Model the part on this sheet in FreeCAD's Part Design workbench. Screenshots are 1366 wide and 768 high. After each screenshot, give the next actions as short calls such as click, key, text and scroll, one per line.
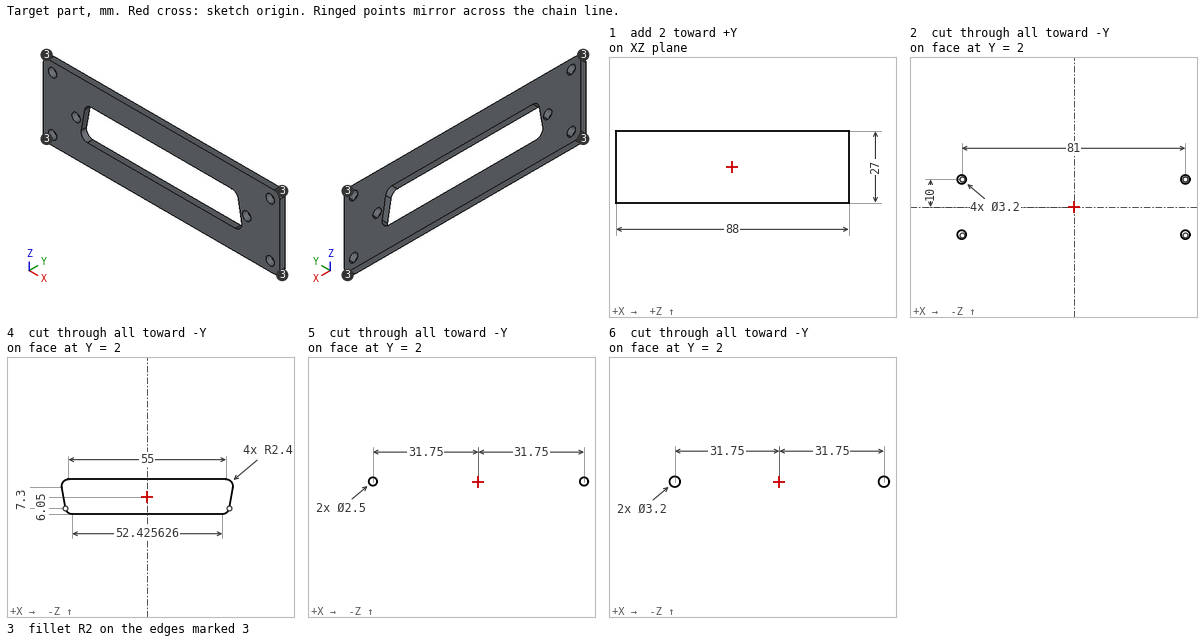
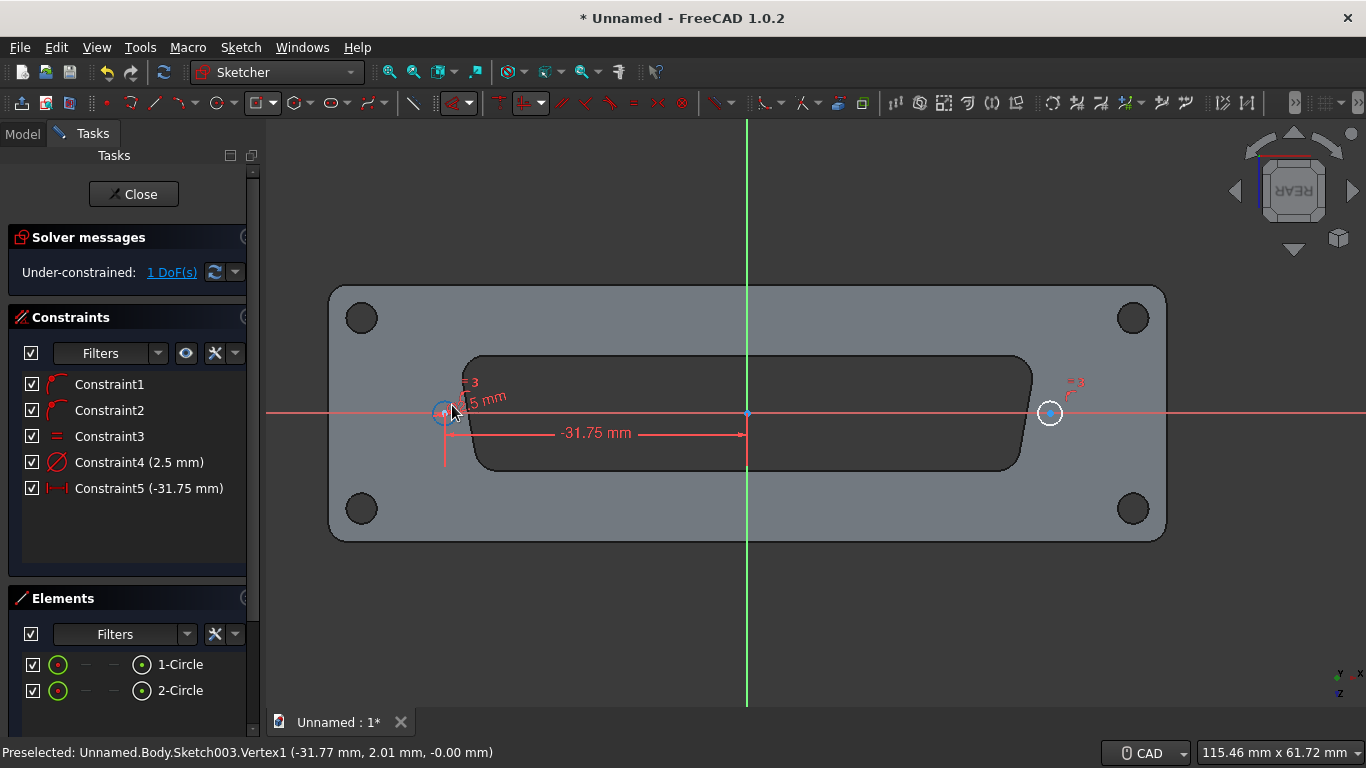
click(1050, 413)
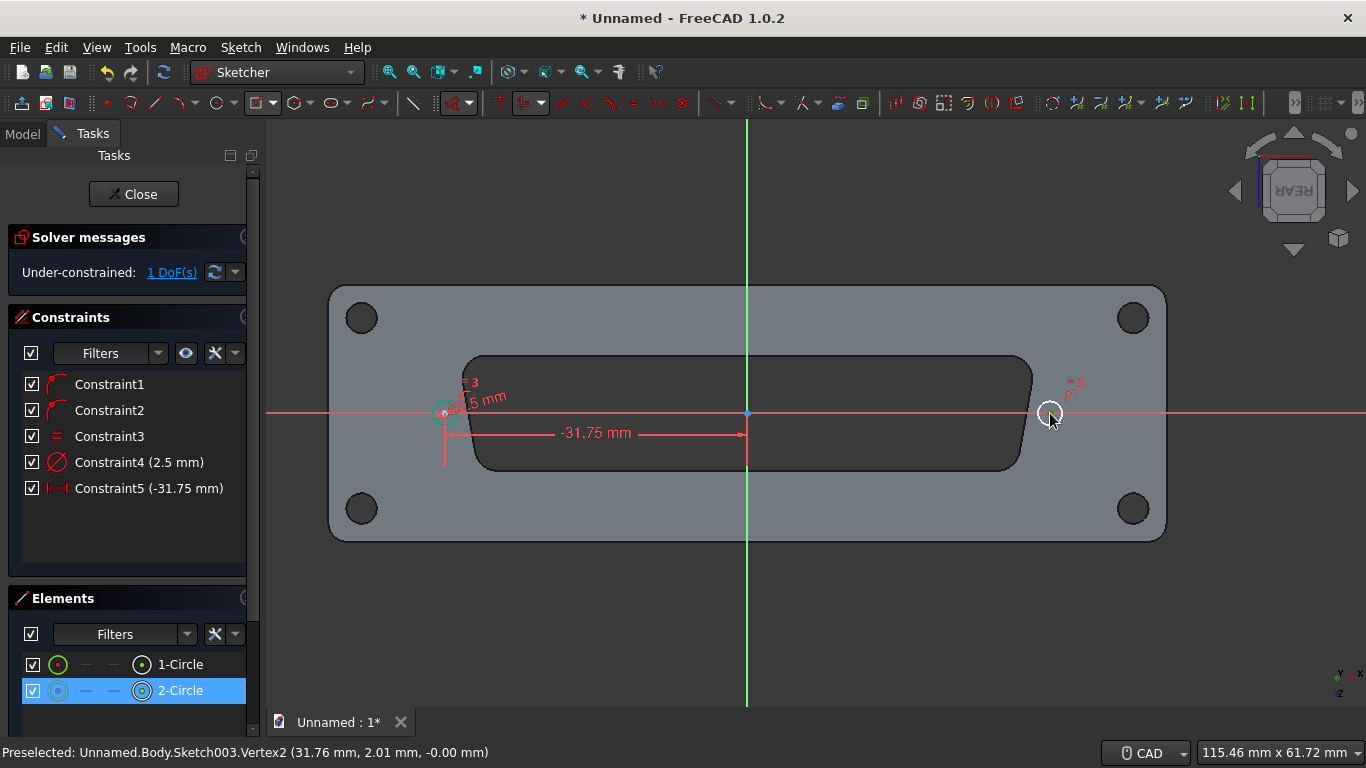
click(472, 104)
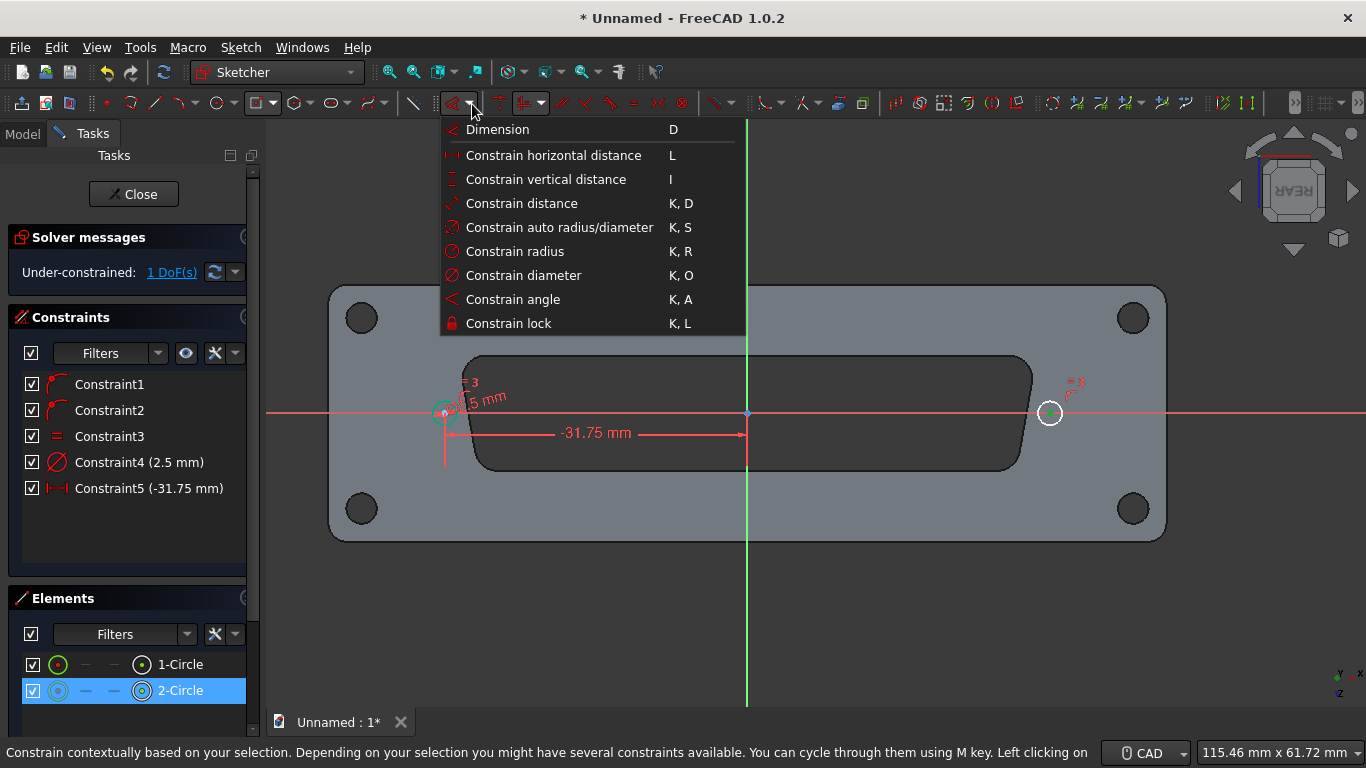
click(593, 155)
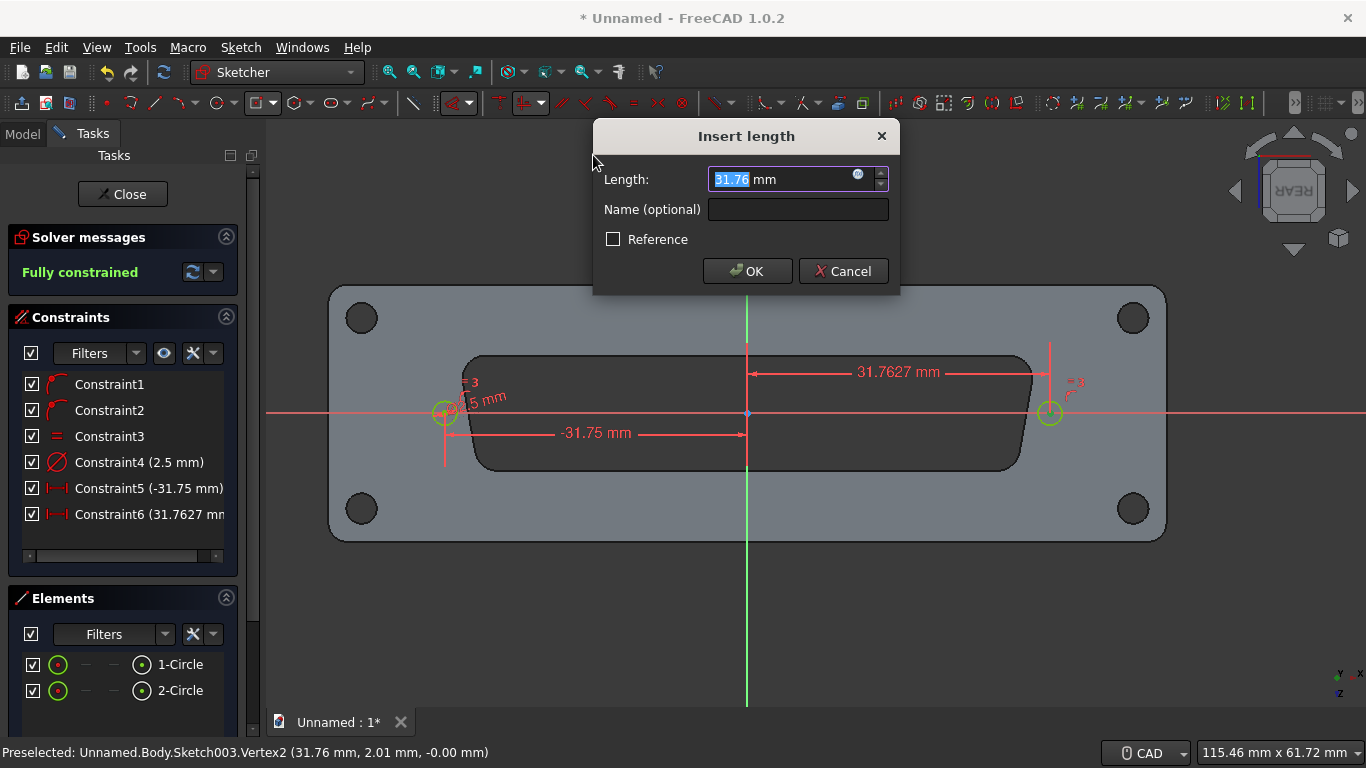
text(31.75)
key(Return)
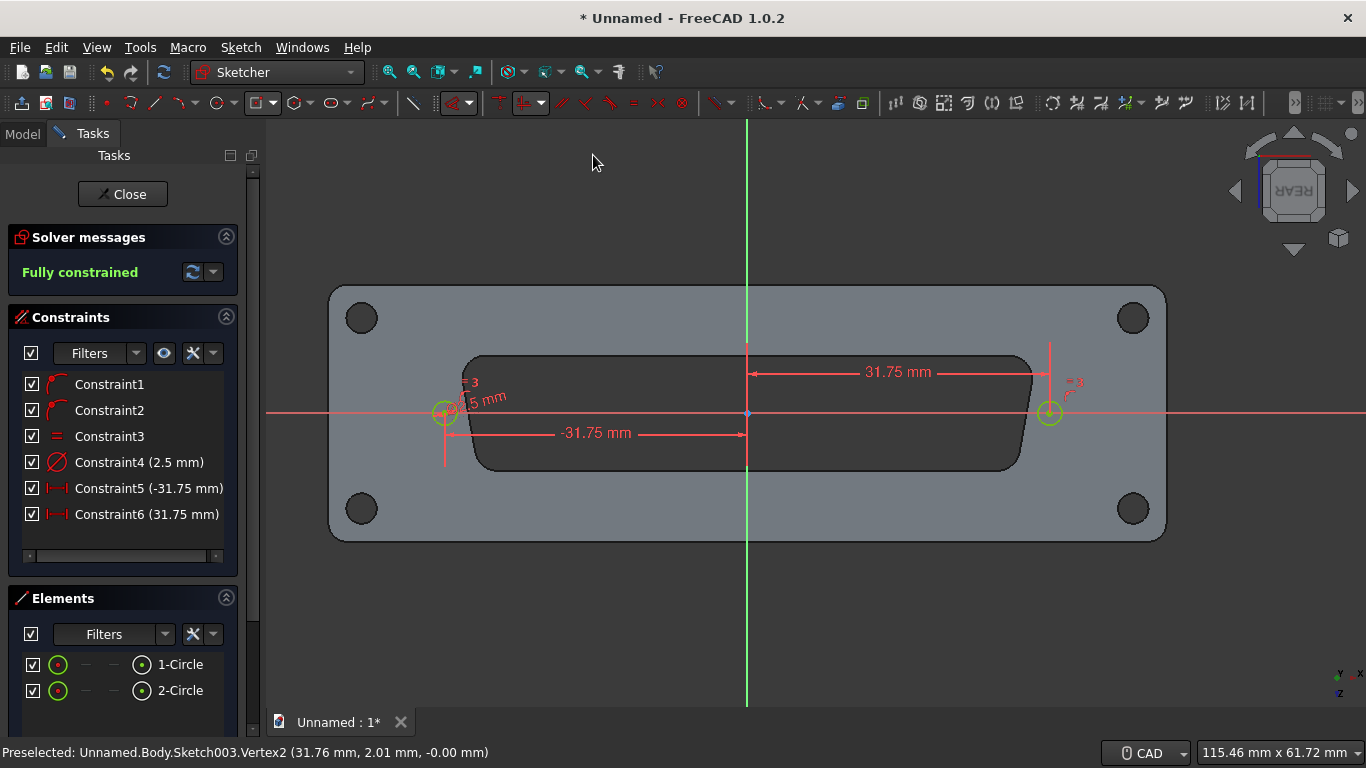
click(123, 194)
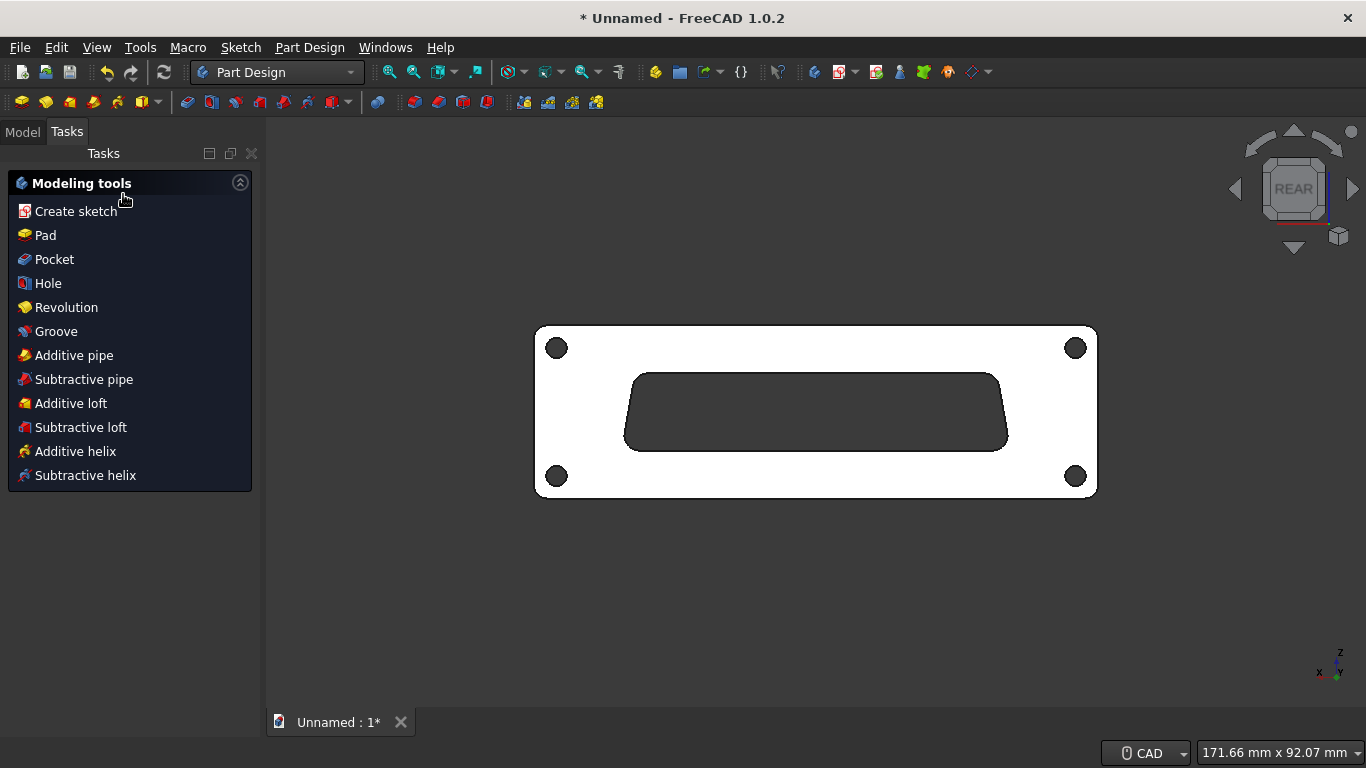
click(188, 102)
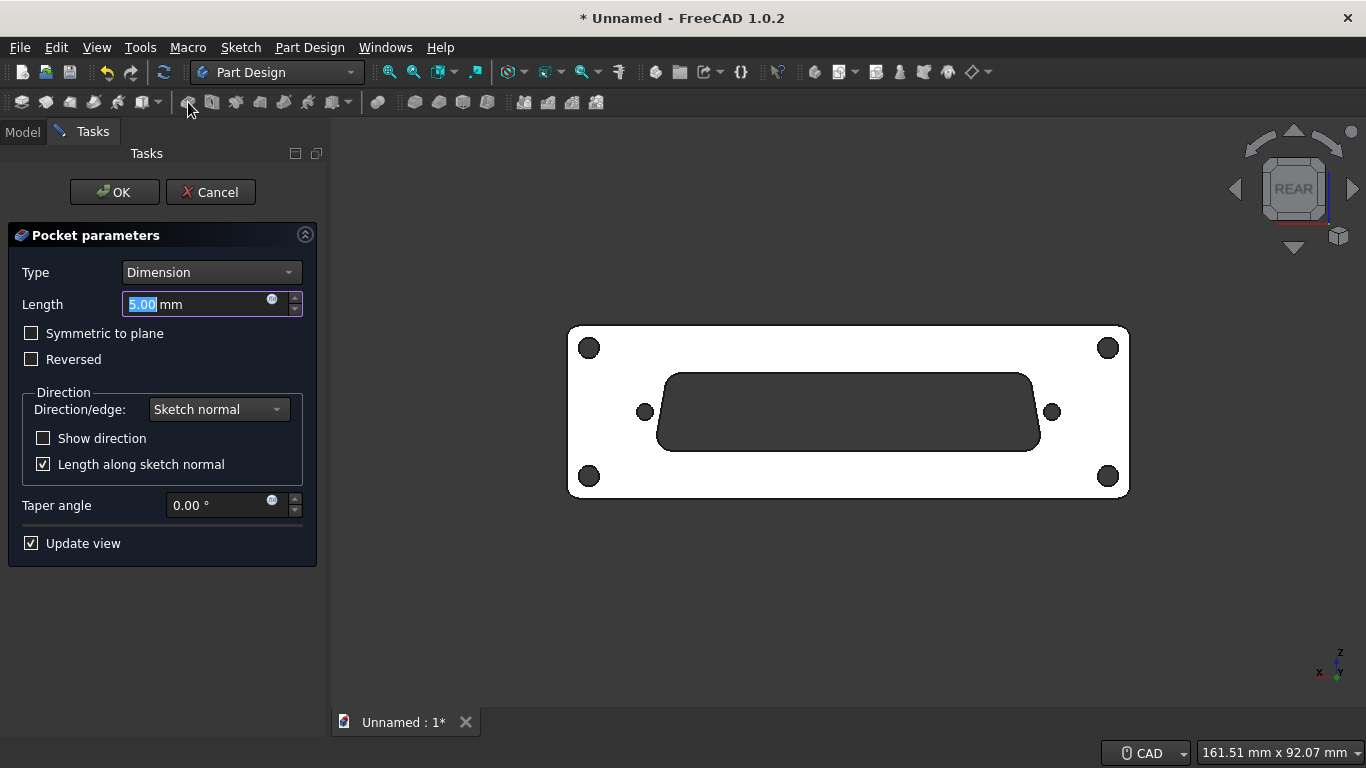
click(212, 272)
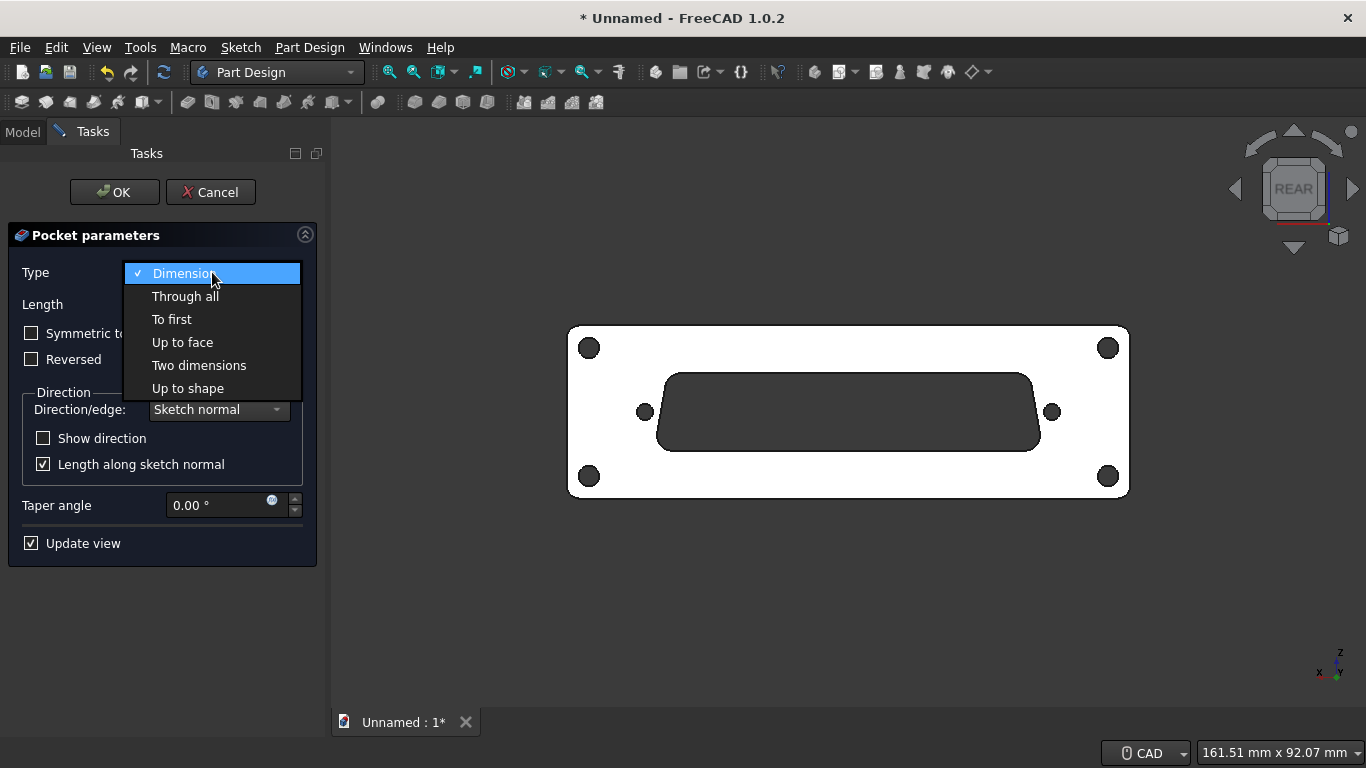
click(212, 296)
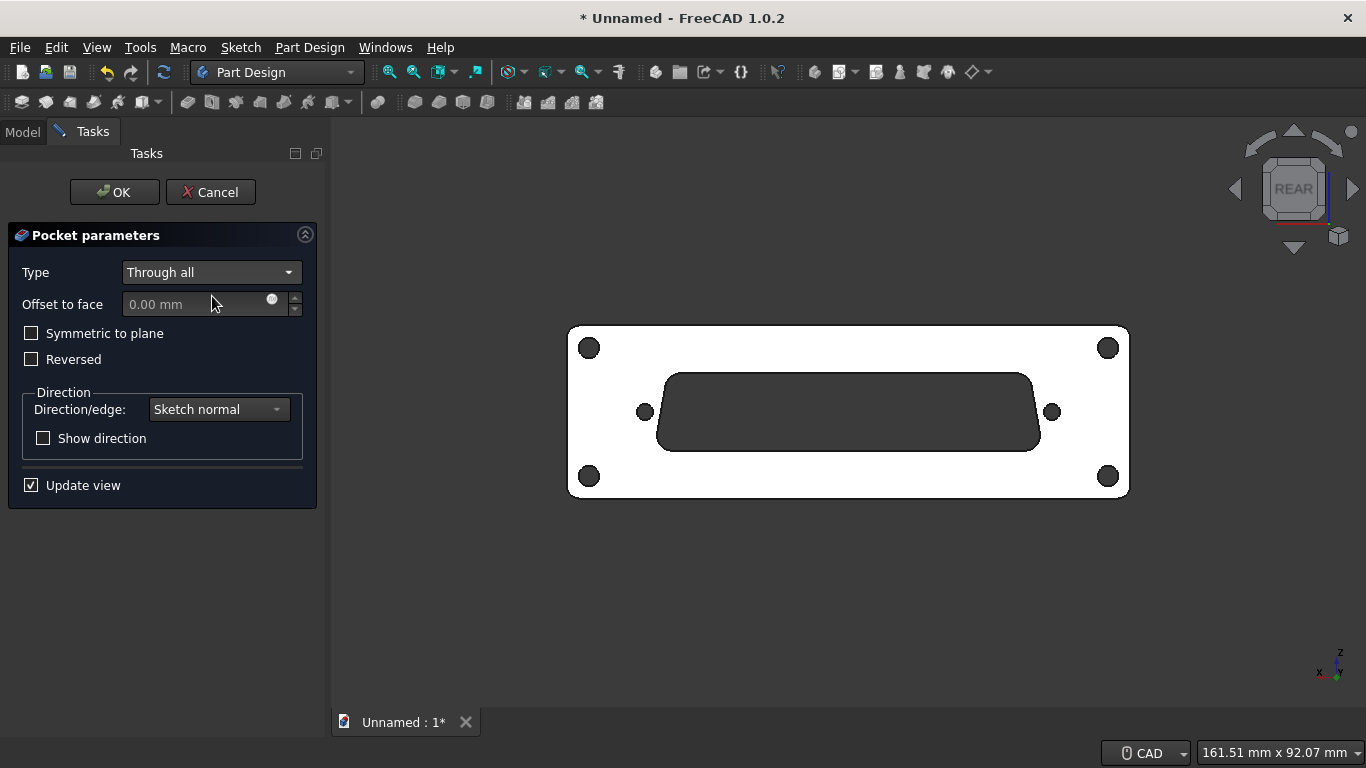
click(115, 192)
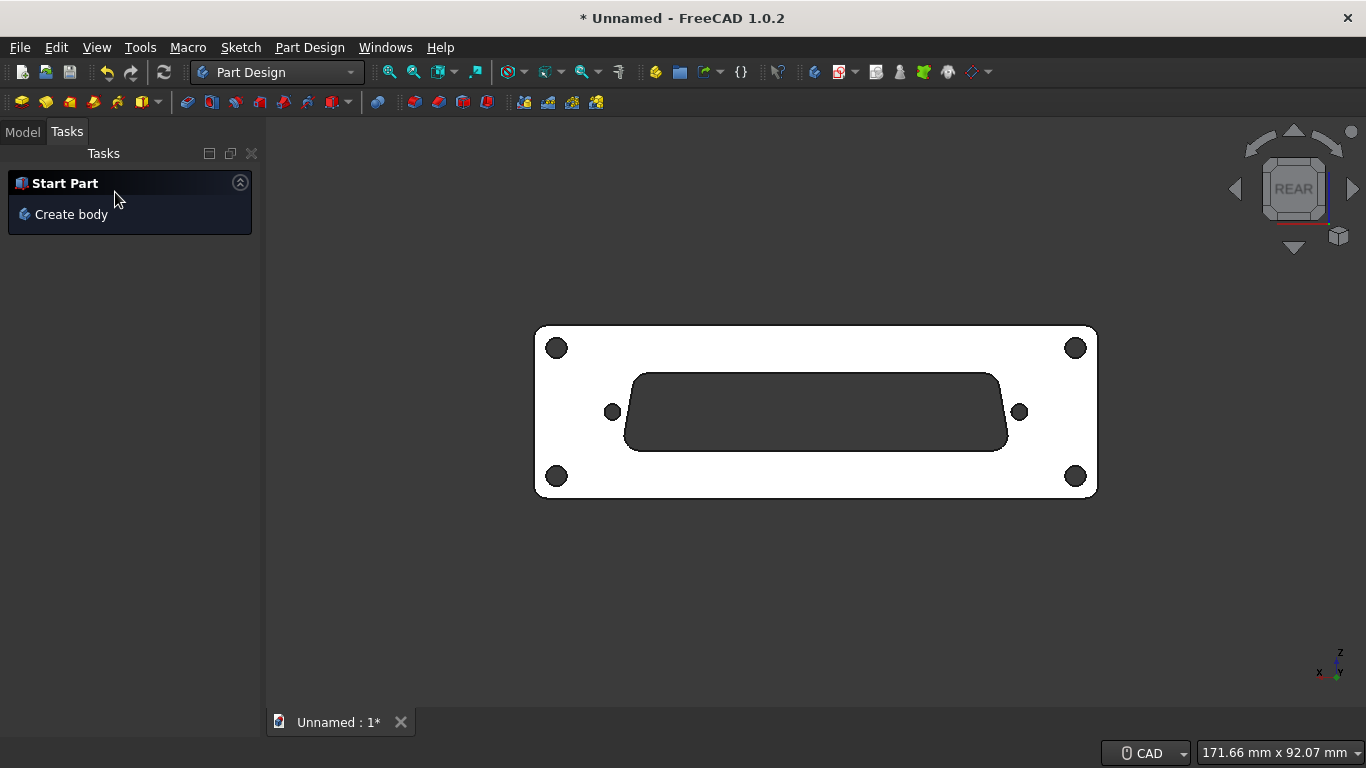
click(574, 386)